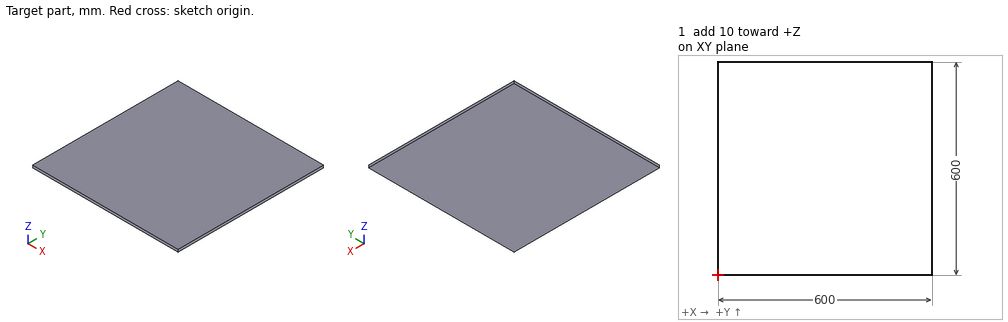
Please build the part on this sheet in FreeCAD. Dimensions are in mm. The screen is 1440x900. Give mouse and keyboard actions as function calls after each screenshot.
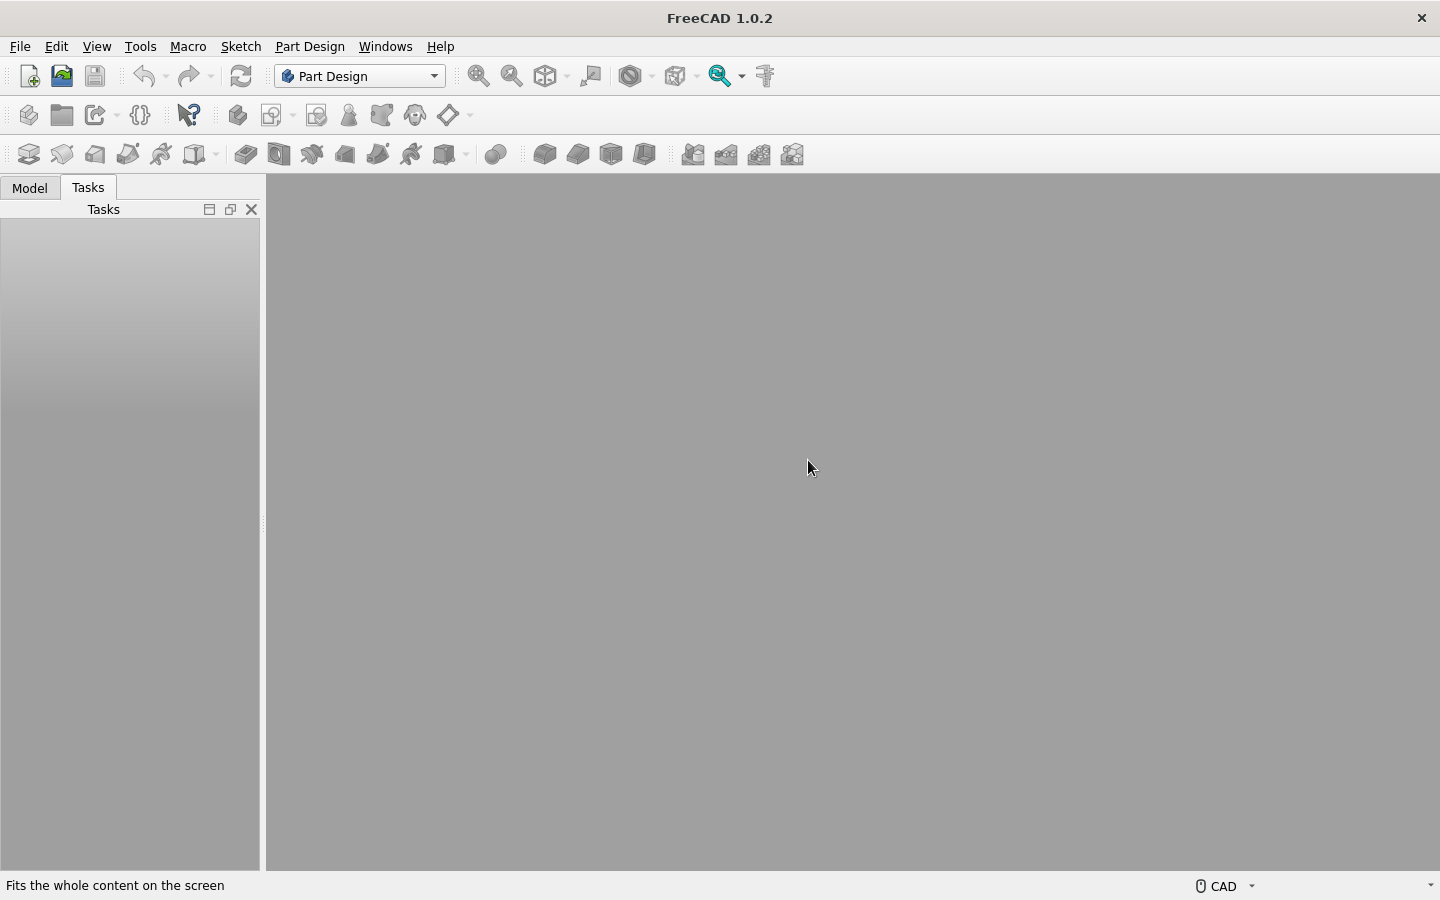
click(29, 76)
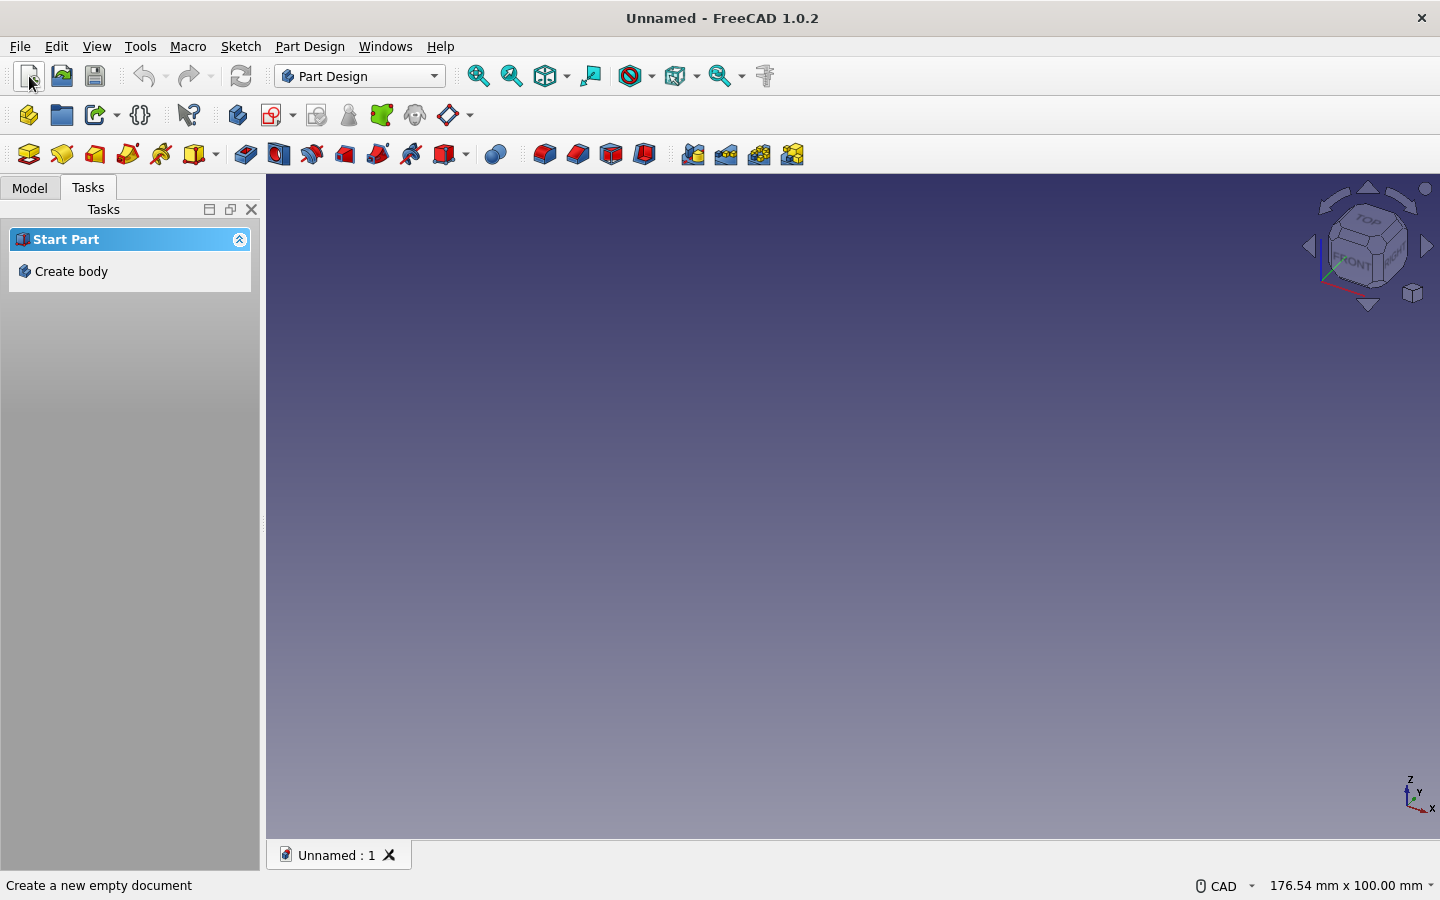
click(270, 116)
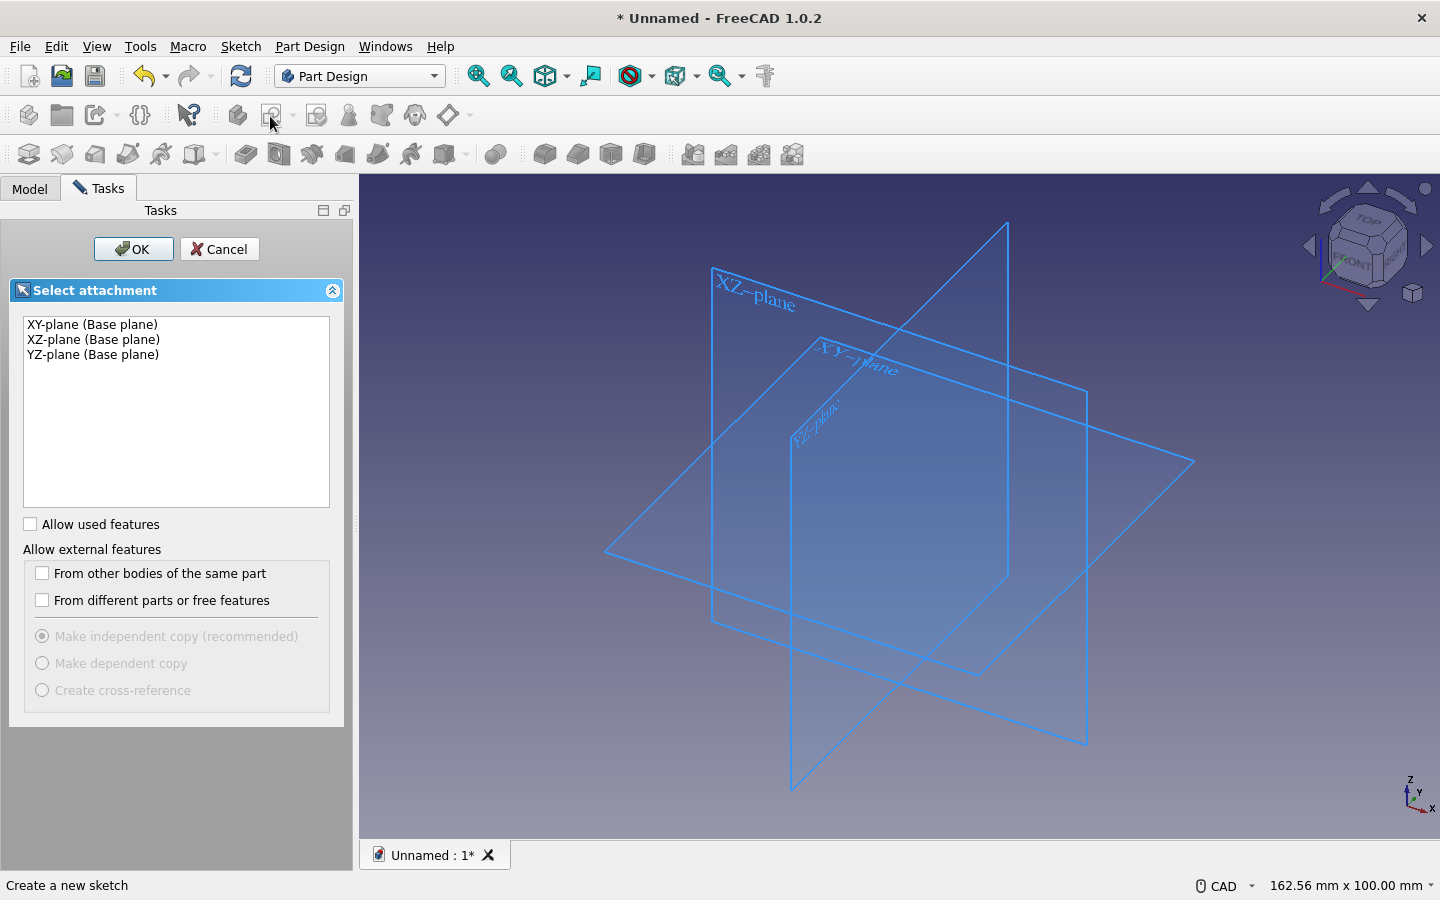
click(84, 324)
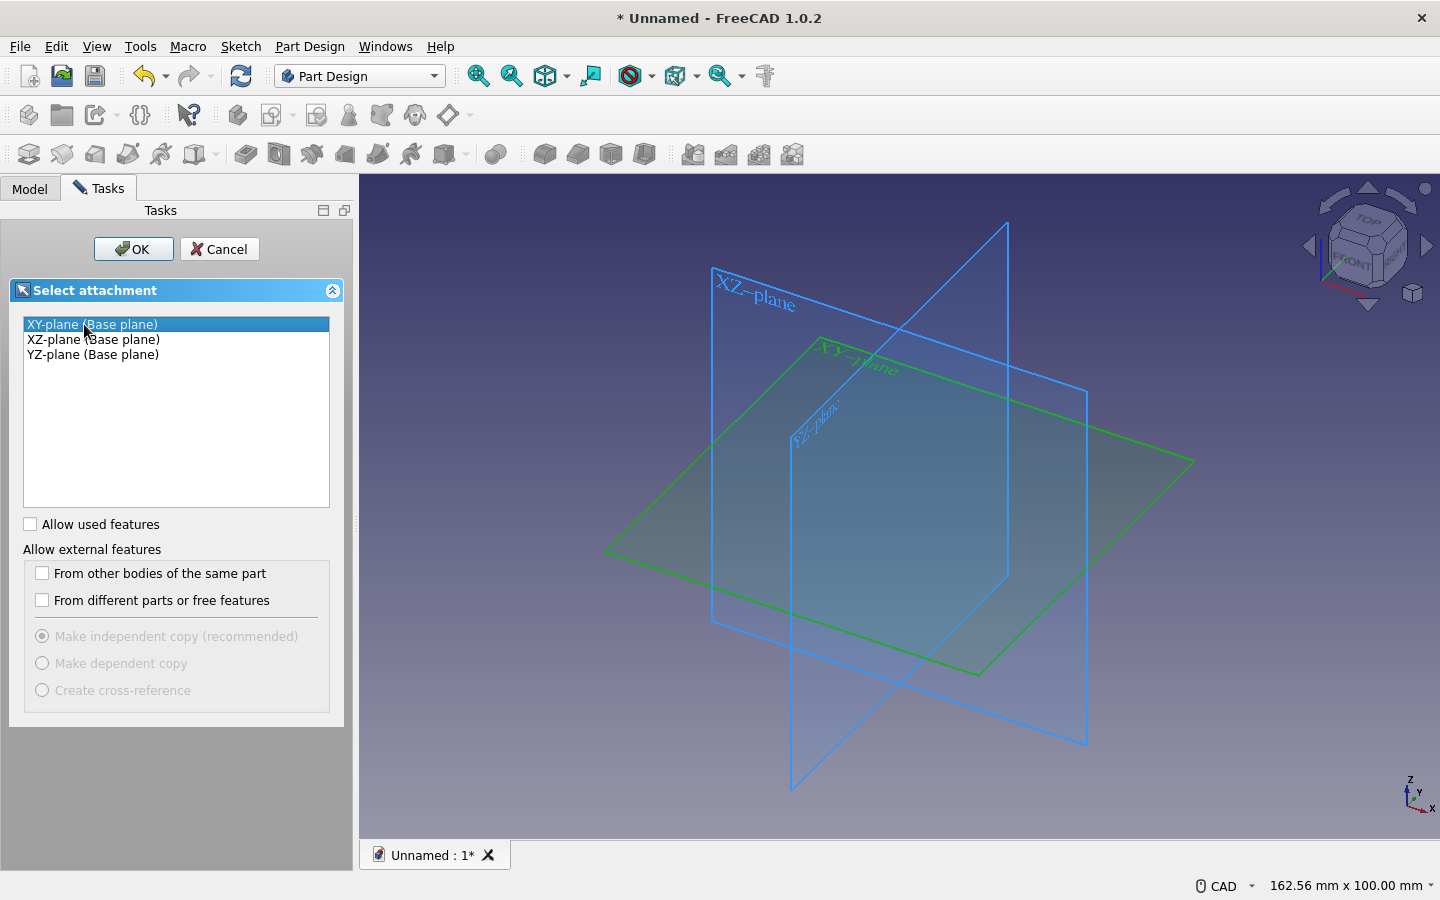
click(134, 249)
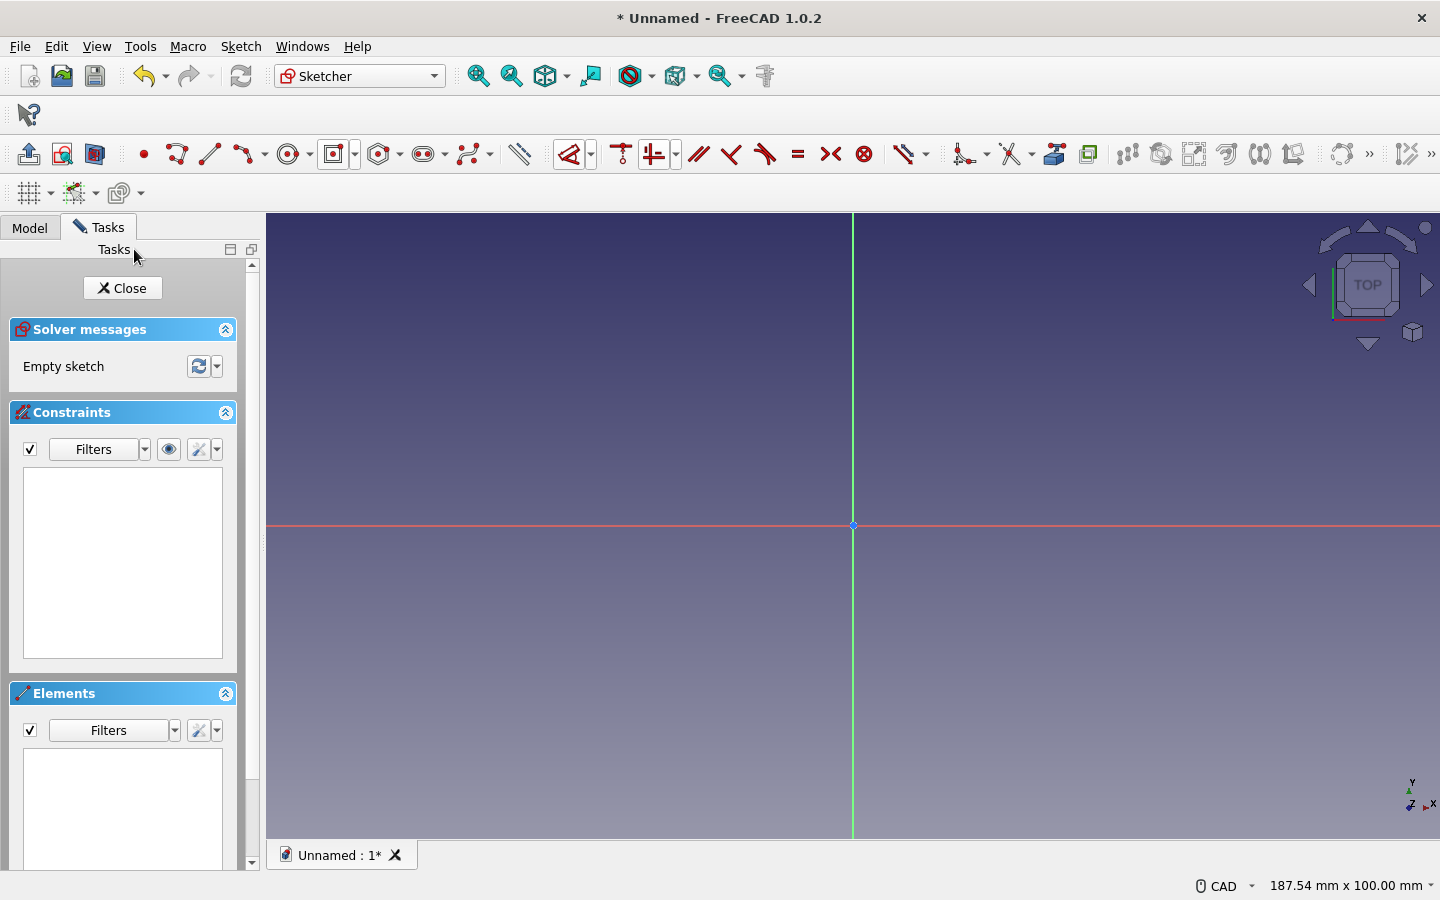
scroll(542, 760, down, 11)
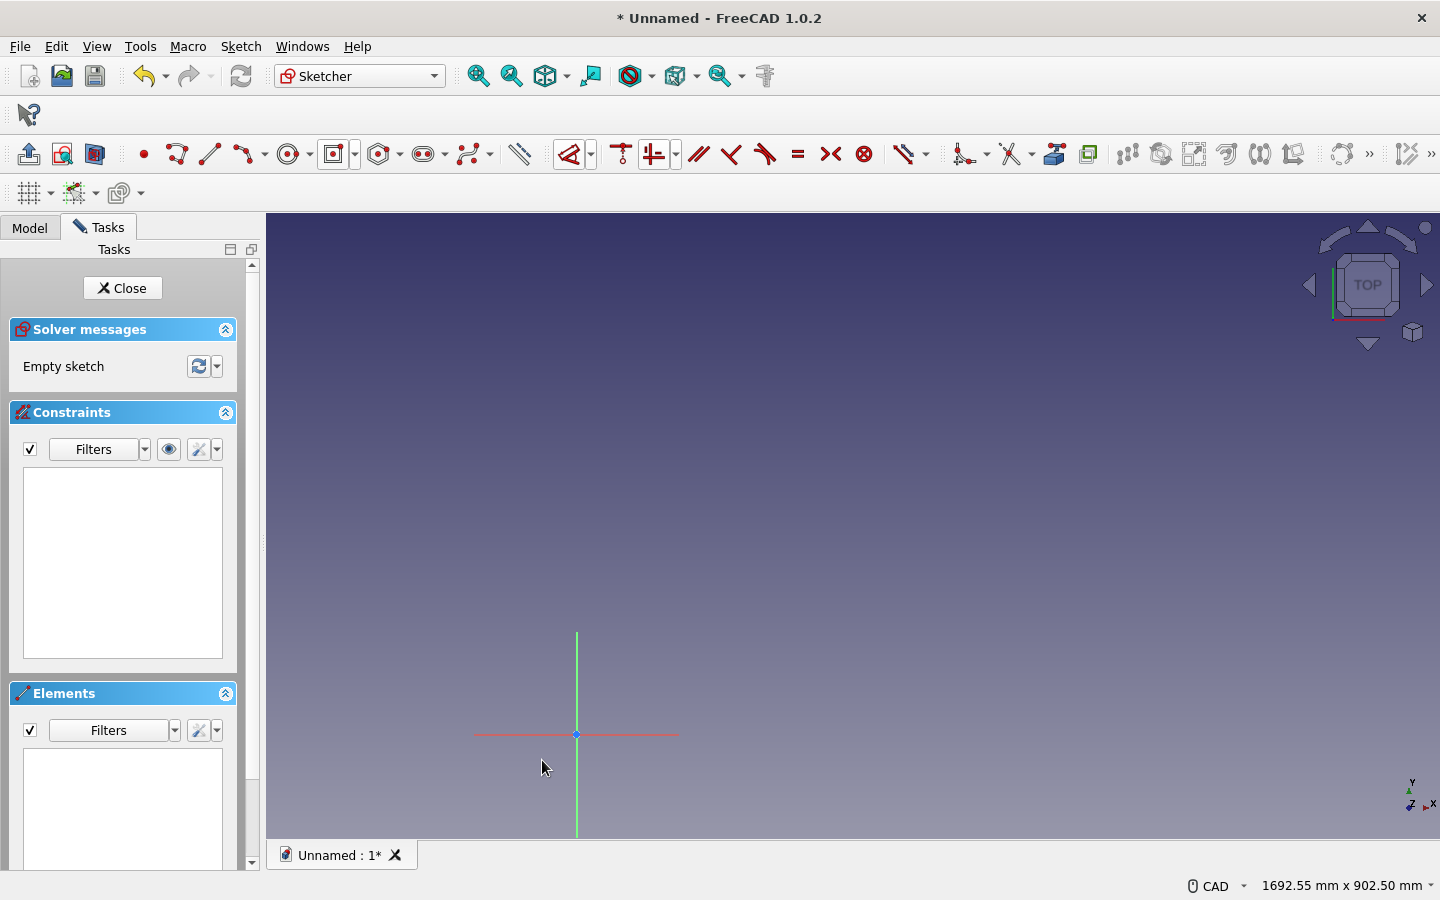
click(354, 154)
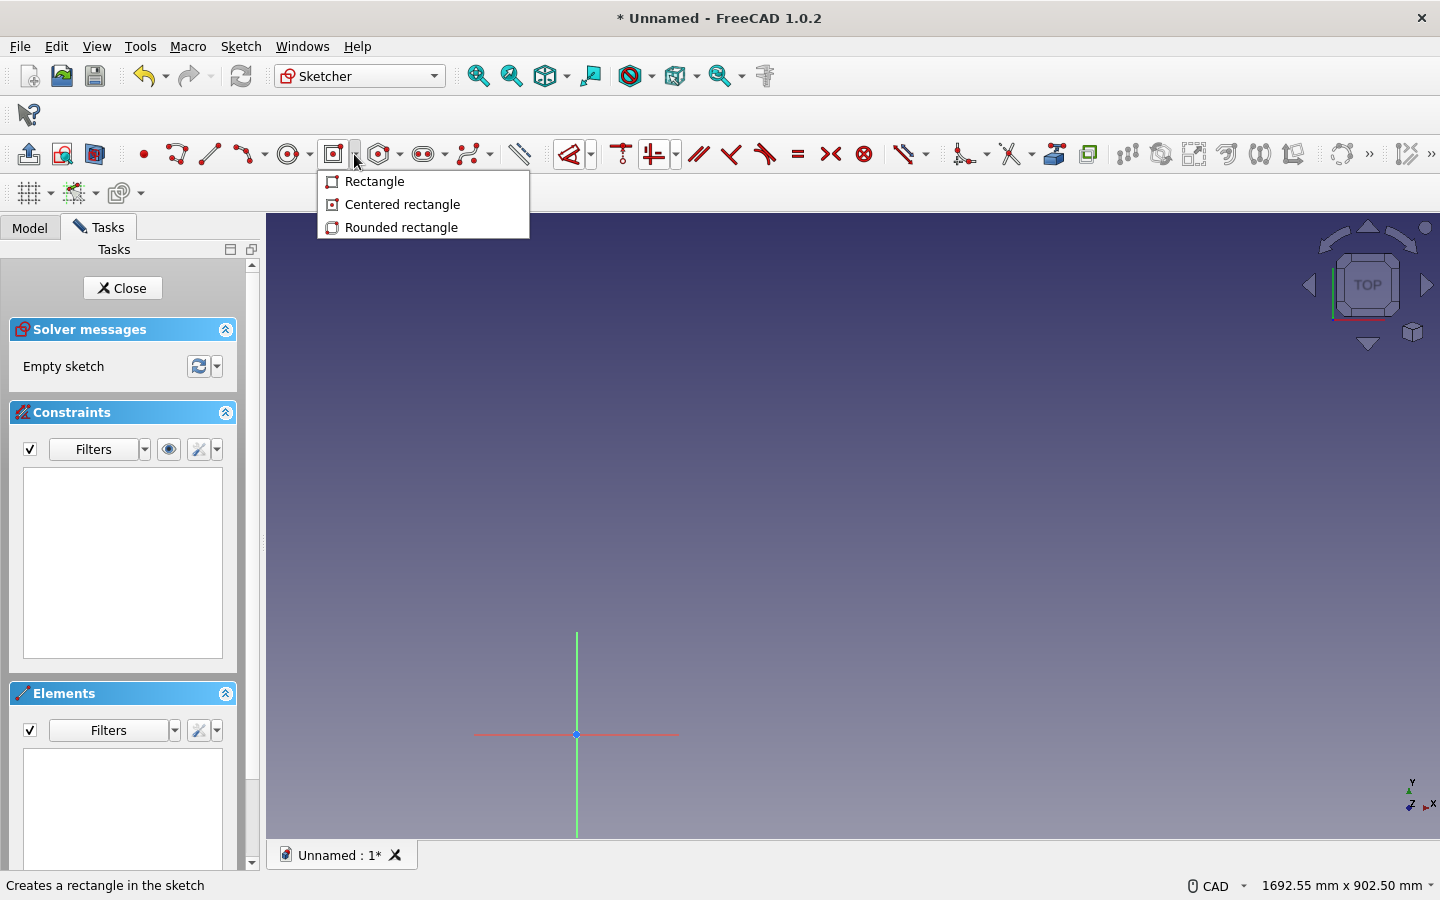
click(424, 182)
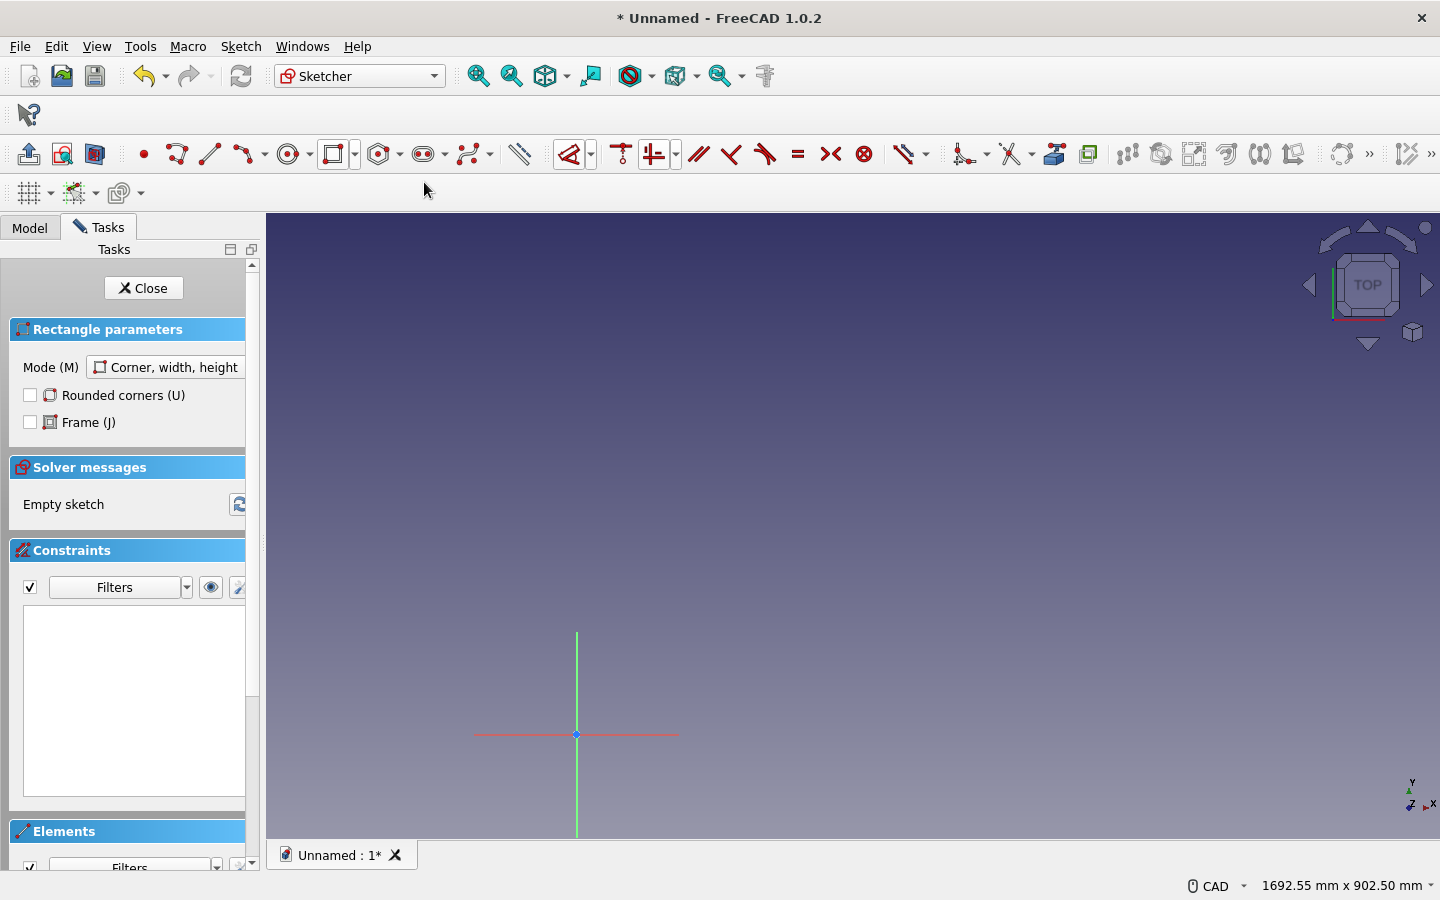
click(577, 735)
click(993, 319)
key(Escape)